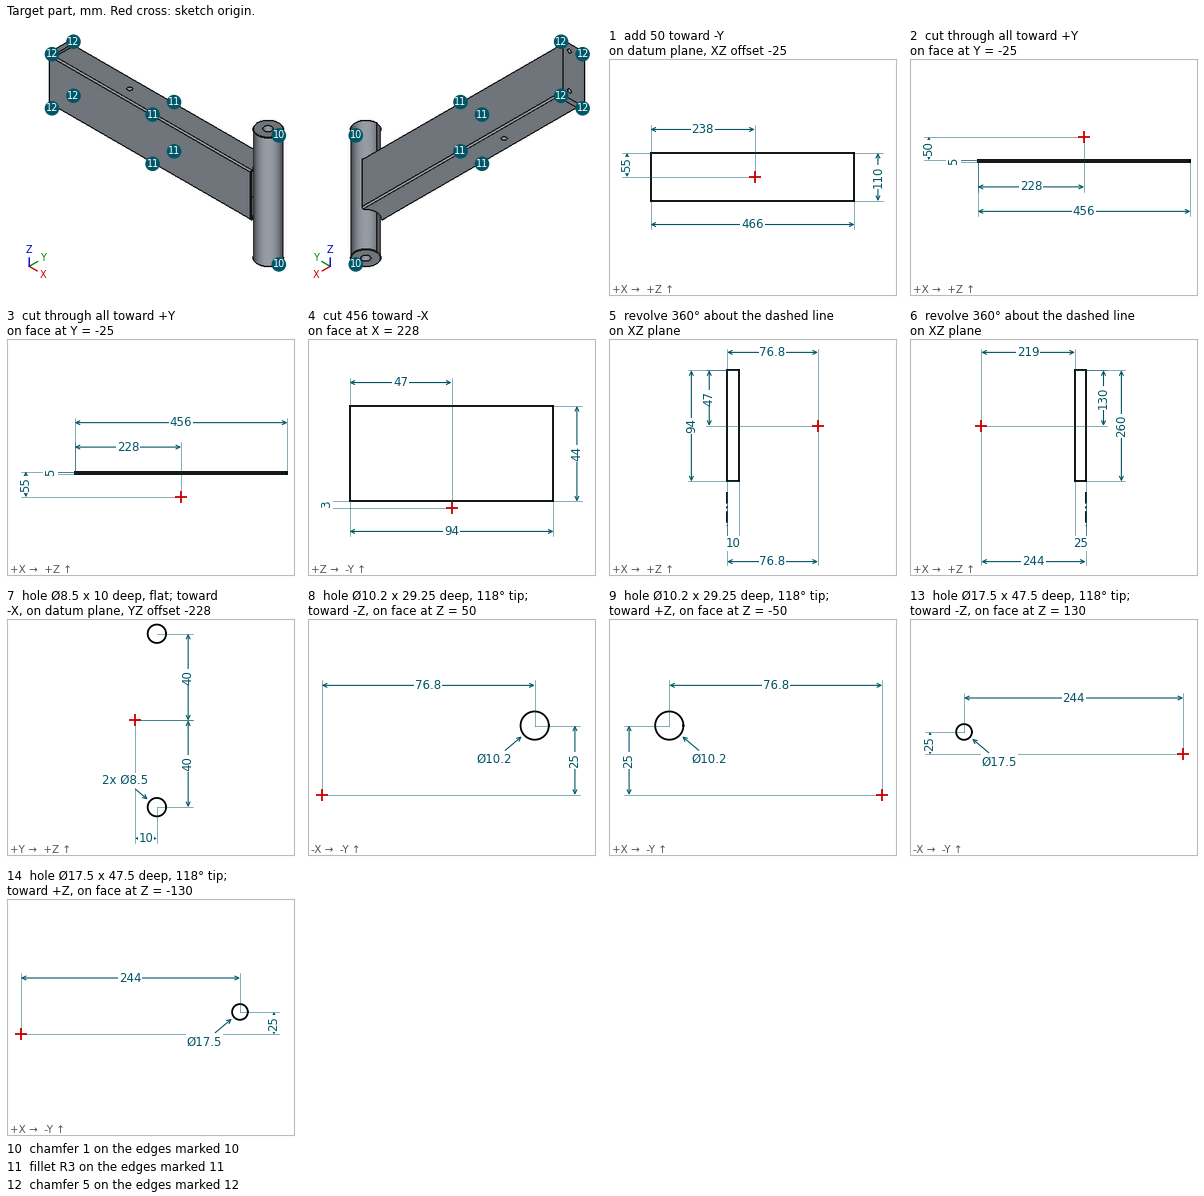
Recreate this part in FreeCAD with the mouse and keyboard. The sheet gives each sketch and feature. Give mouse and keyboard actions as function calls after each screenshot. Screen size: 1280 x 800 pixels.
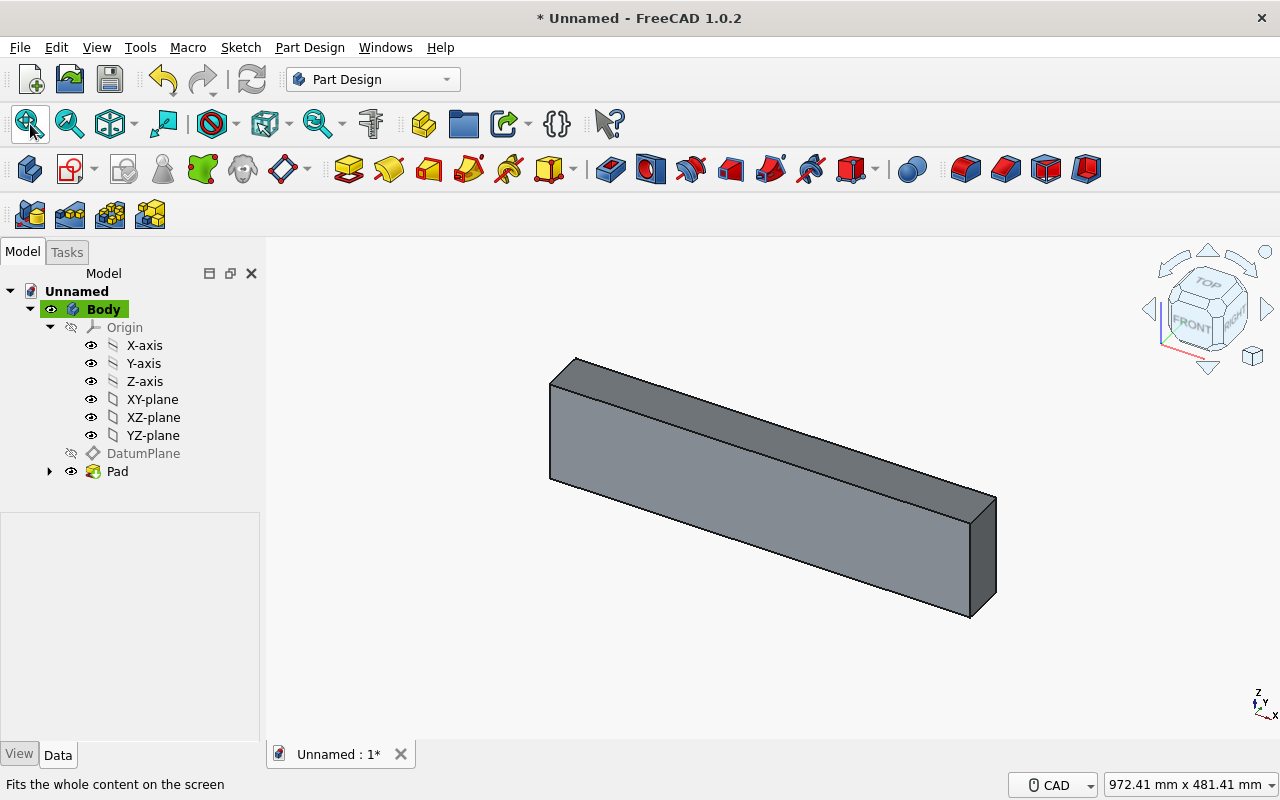
click(880, 540)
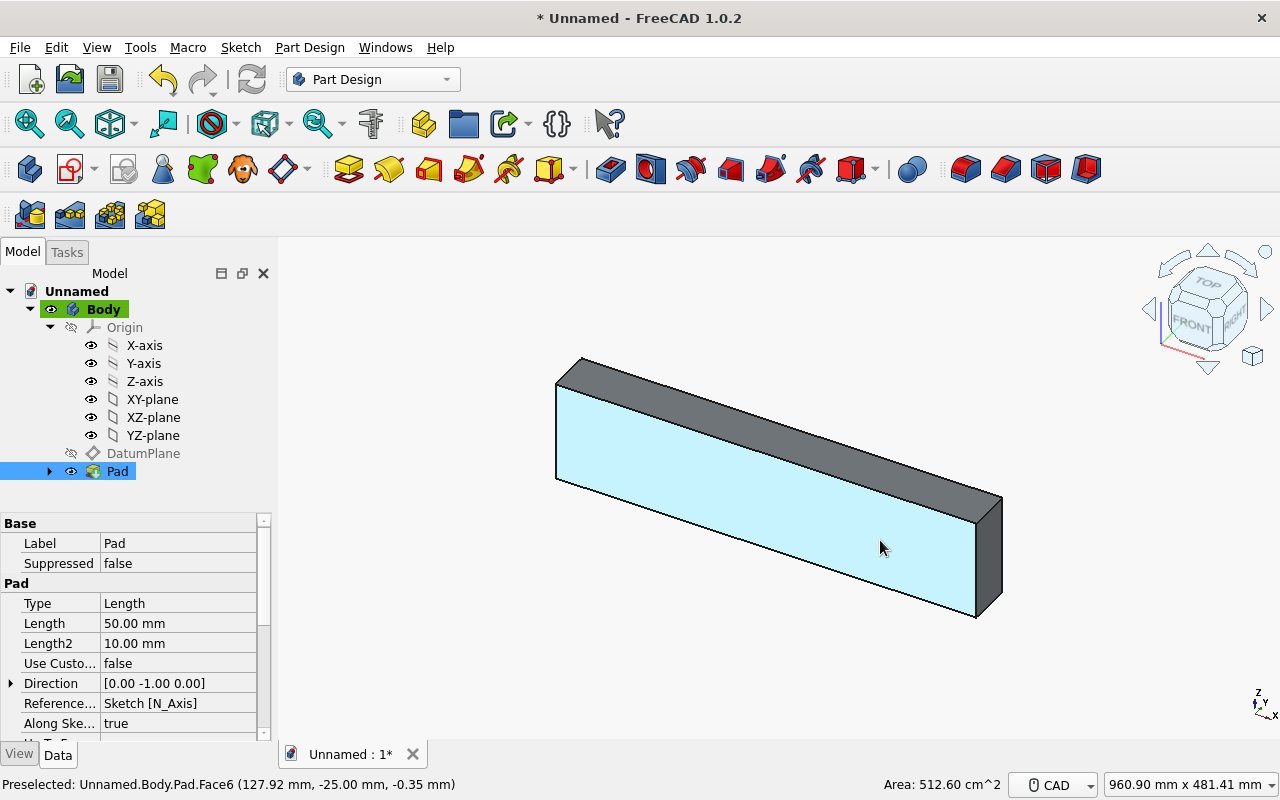
click(70, 170)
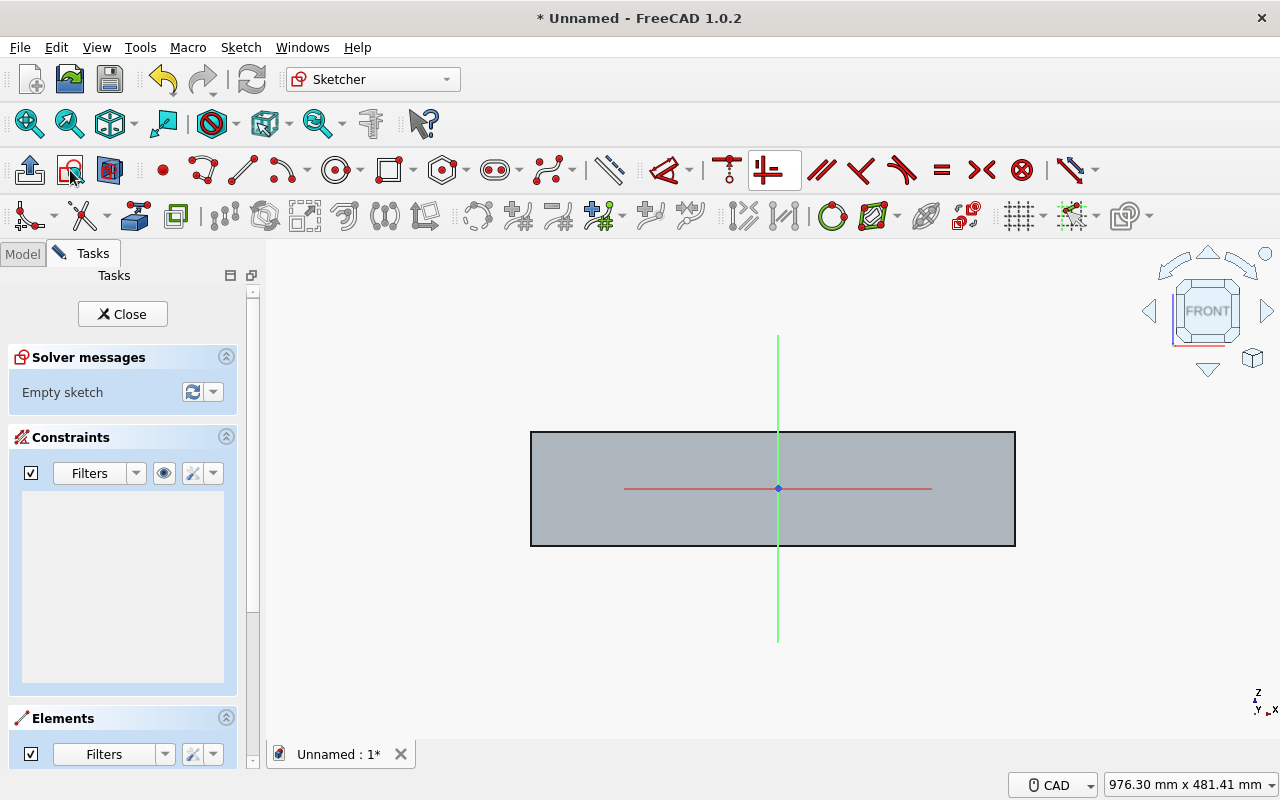
click(390, 170)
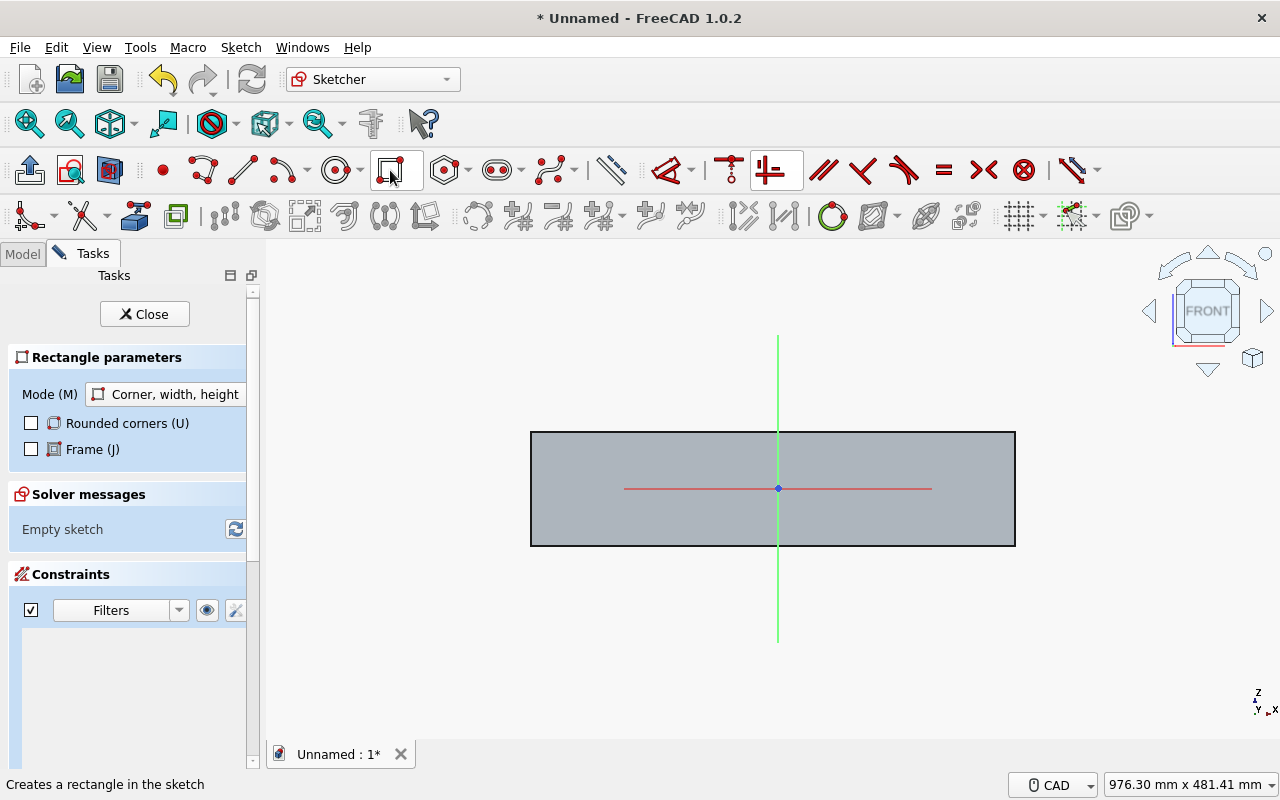
scroll(541, 541, up, 6)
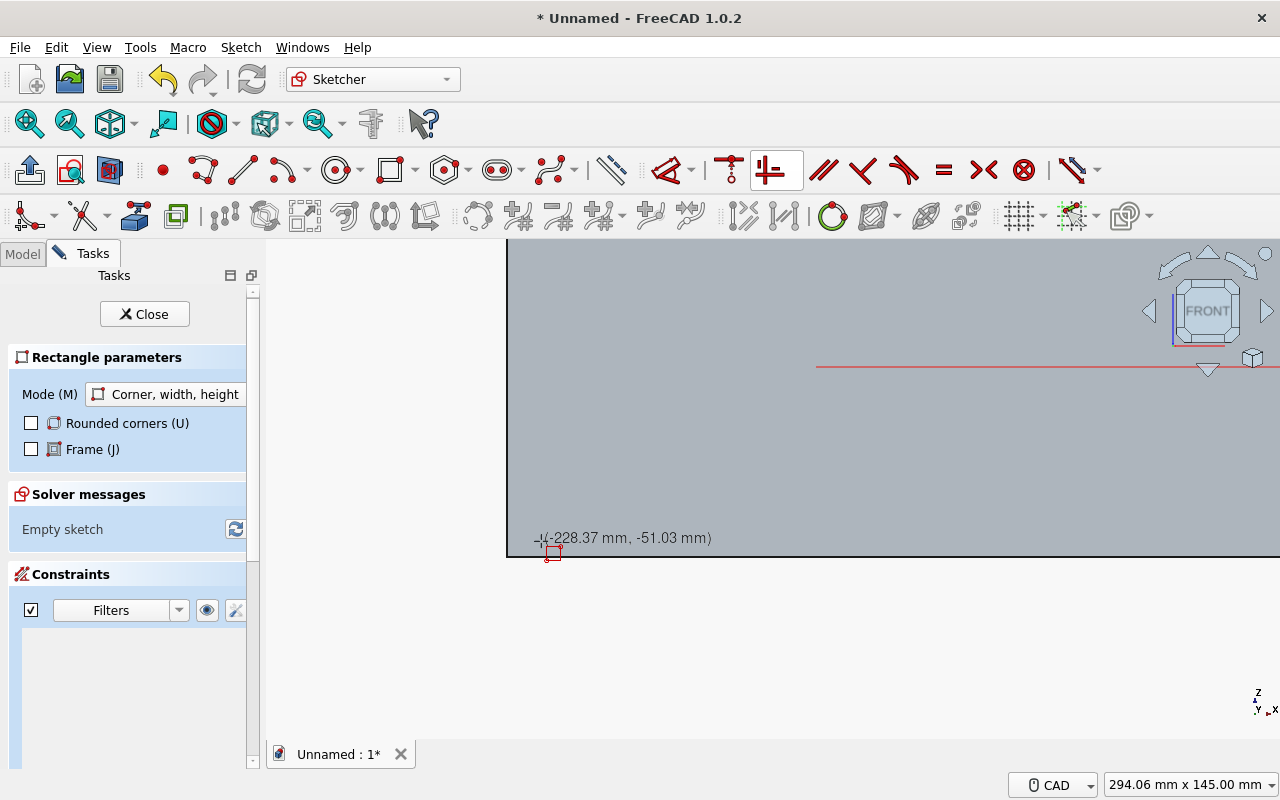
click(542, 539)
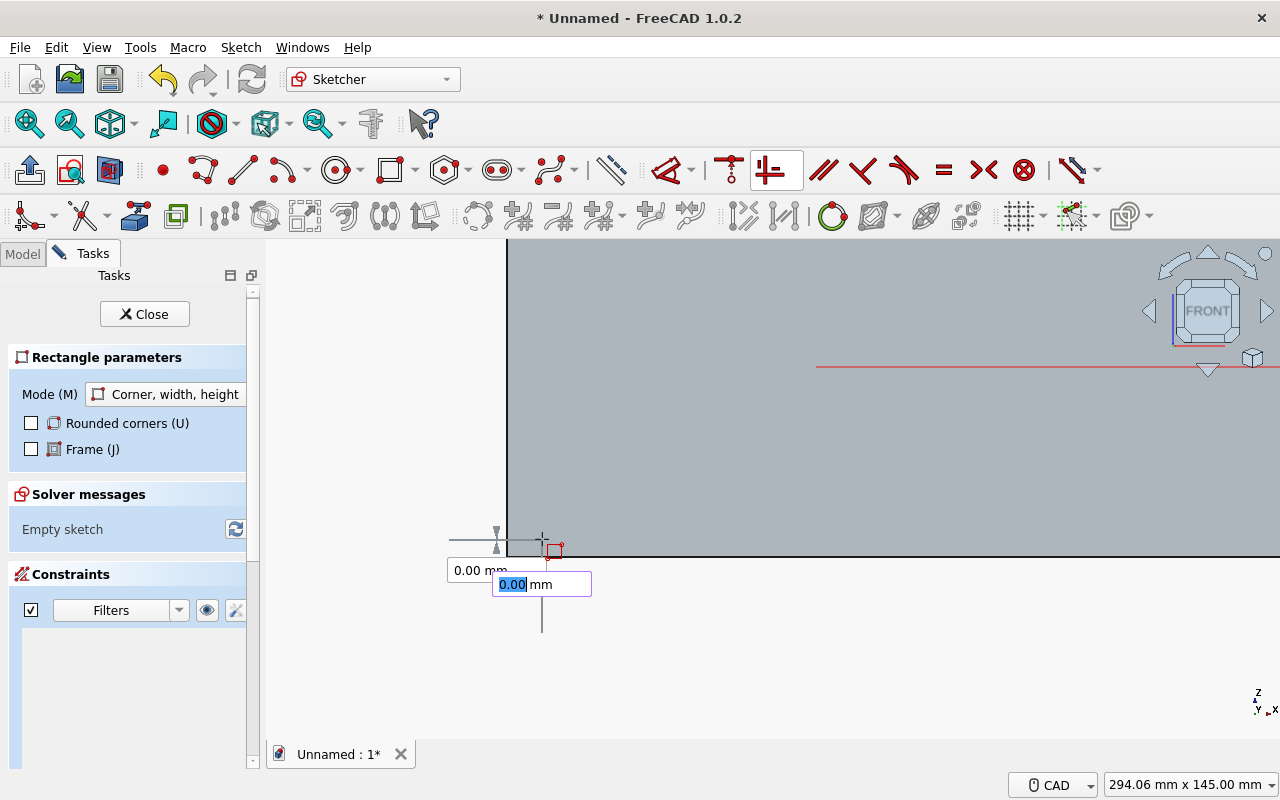
scroll(342, 505, down, 5)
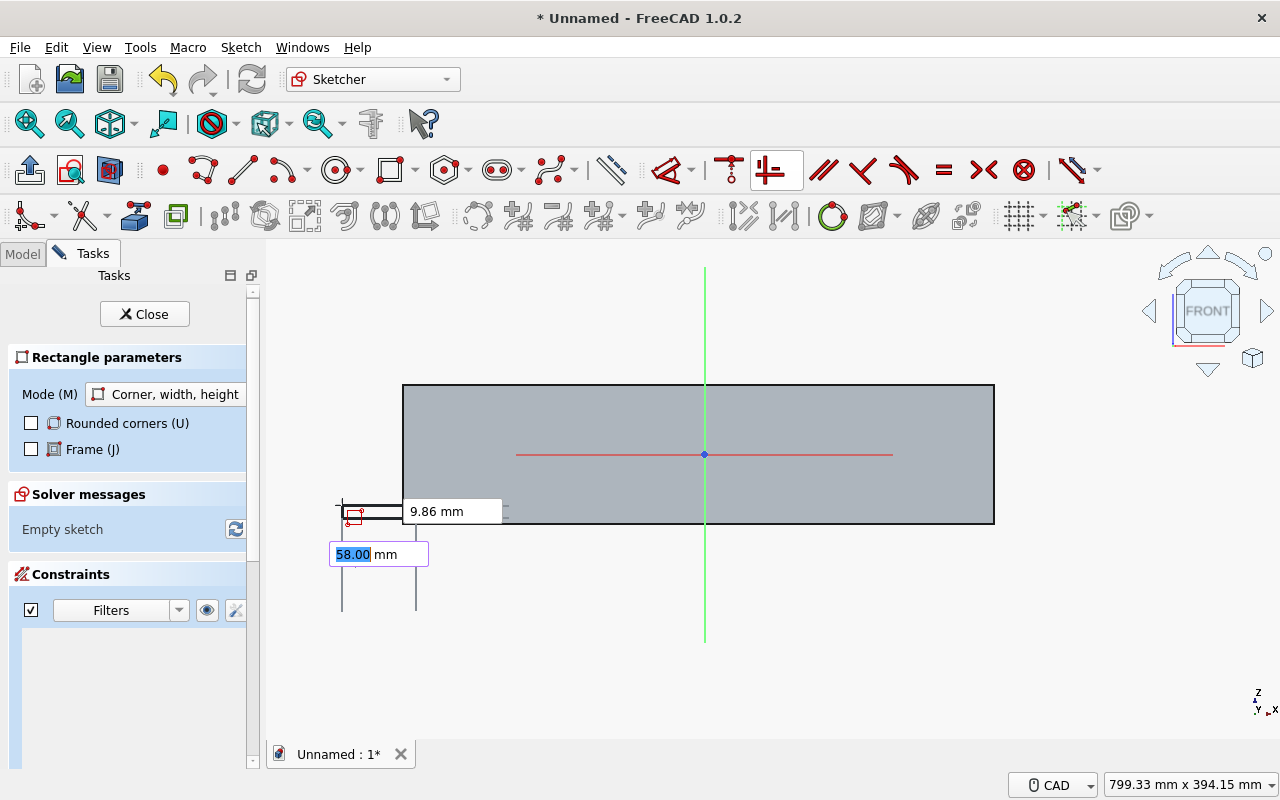
click(994, 524)
key(Escape)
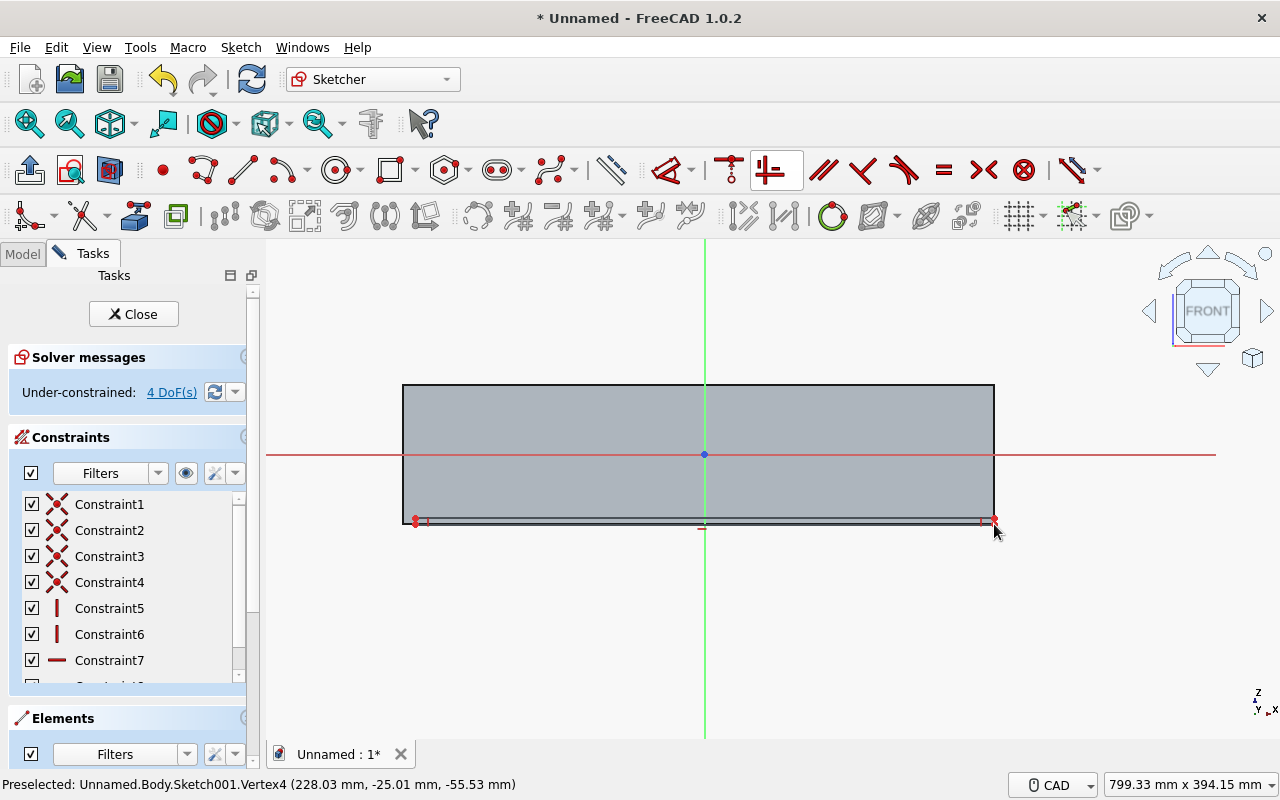
click(666, 170)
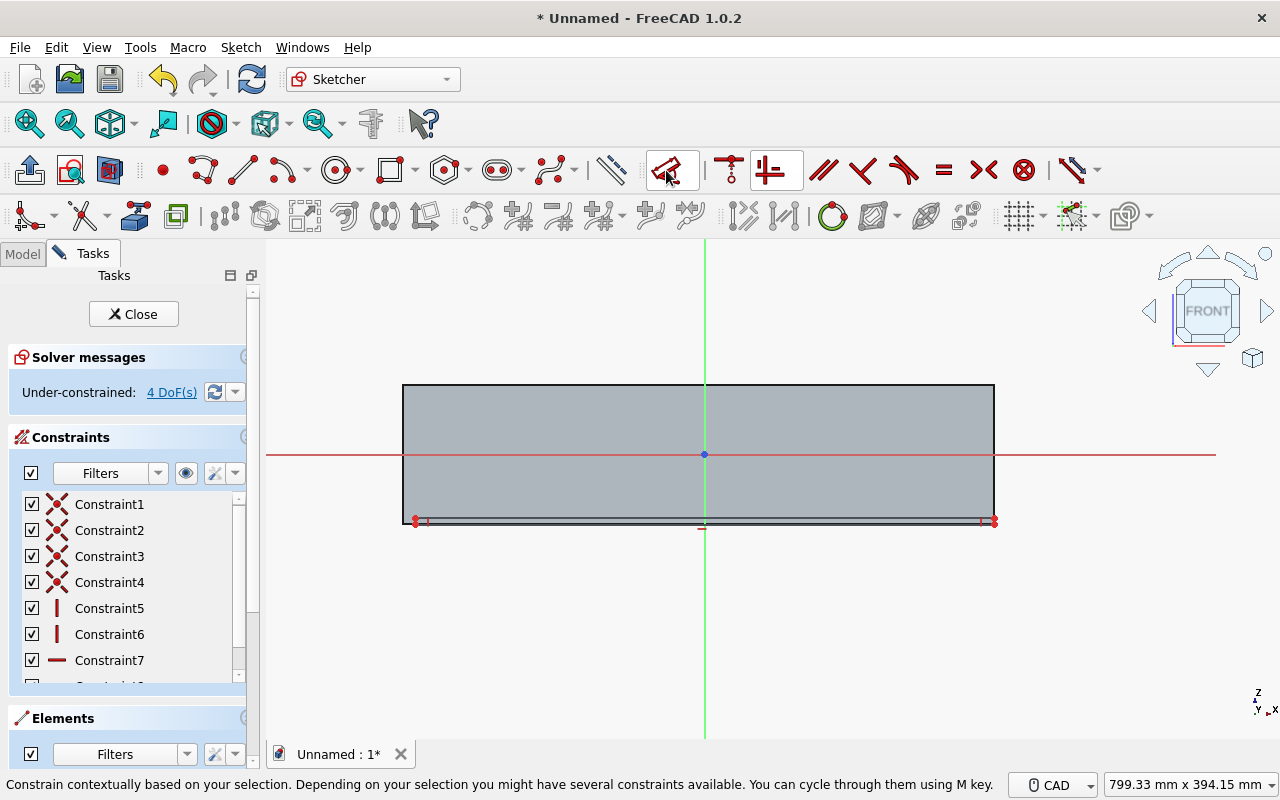
scroll(416, 522, up, 10)